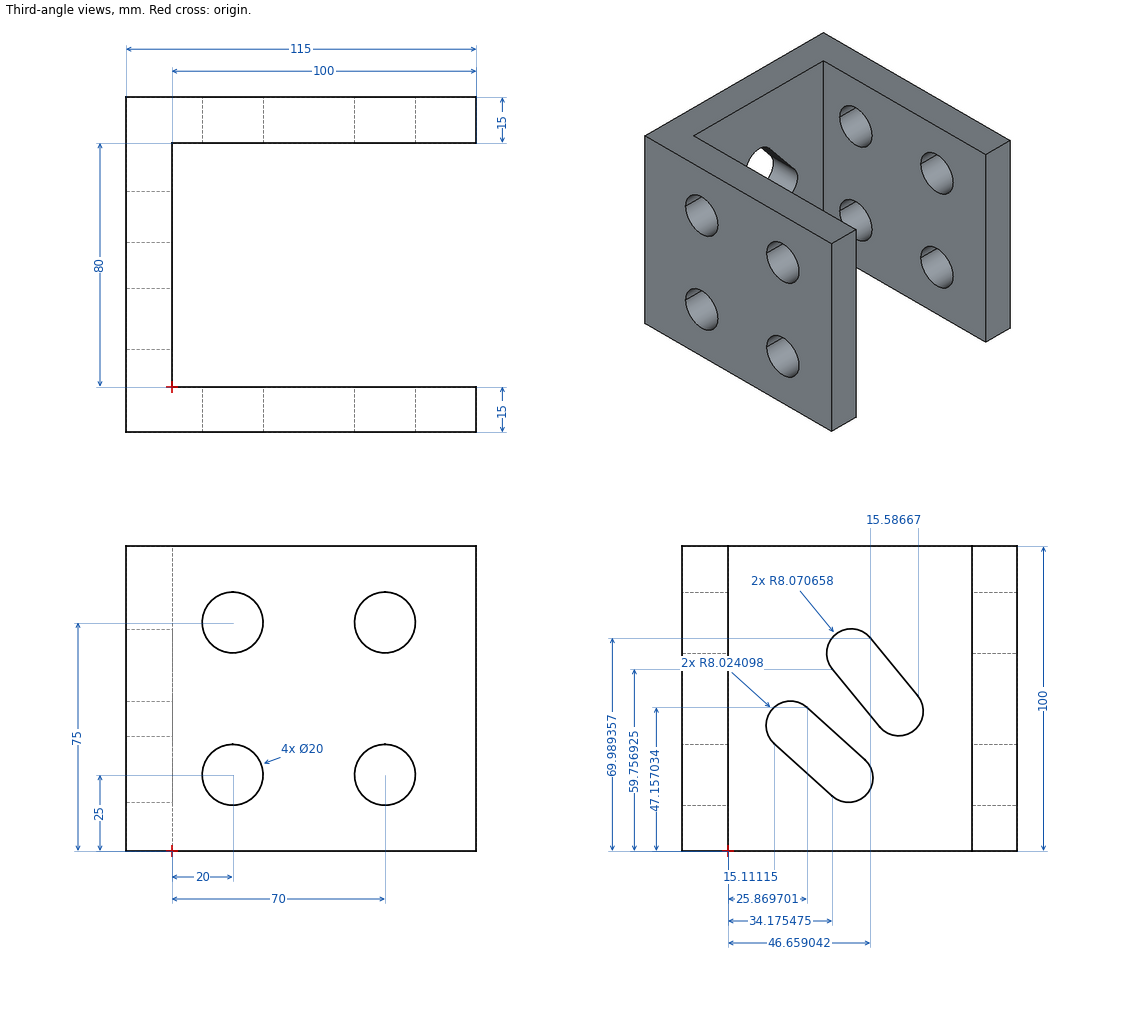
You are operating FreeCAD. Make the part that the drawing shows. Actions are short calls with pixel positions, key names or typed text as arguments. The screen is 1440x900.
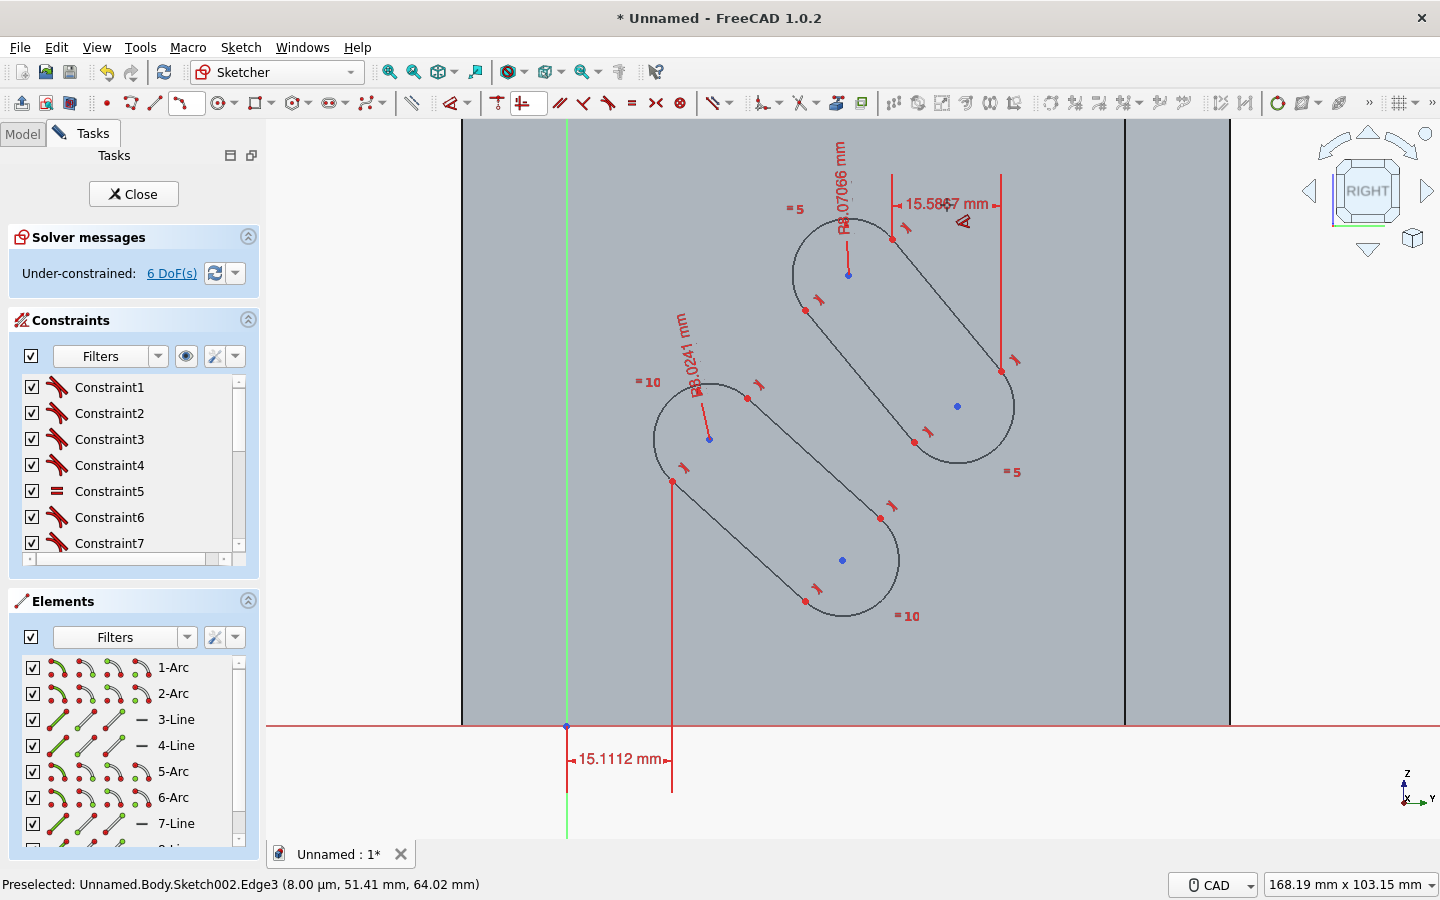
click(892, 239)
click(730, 760)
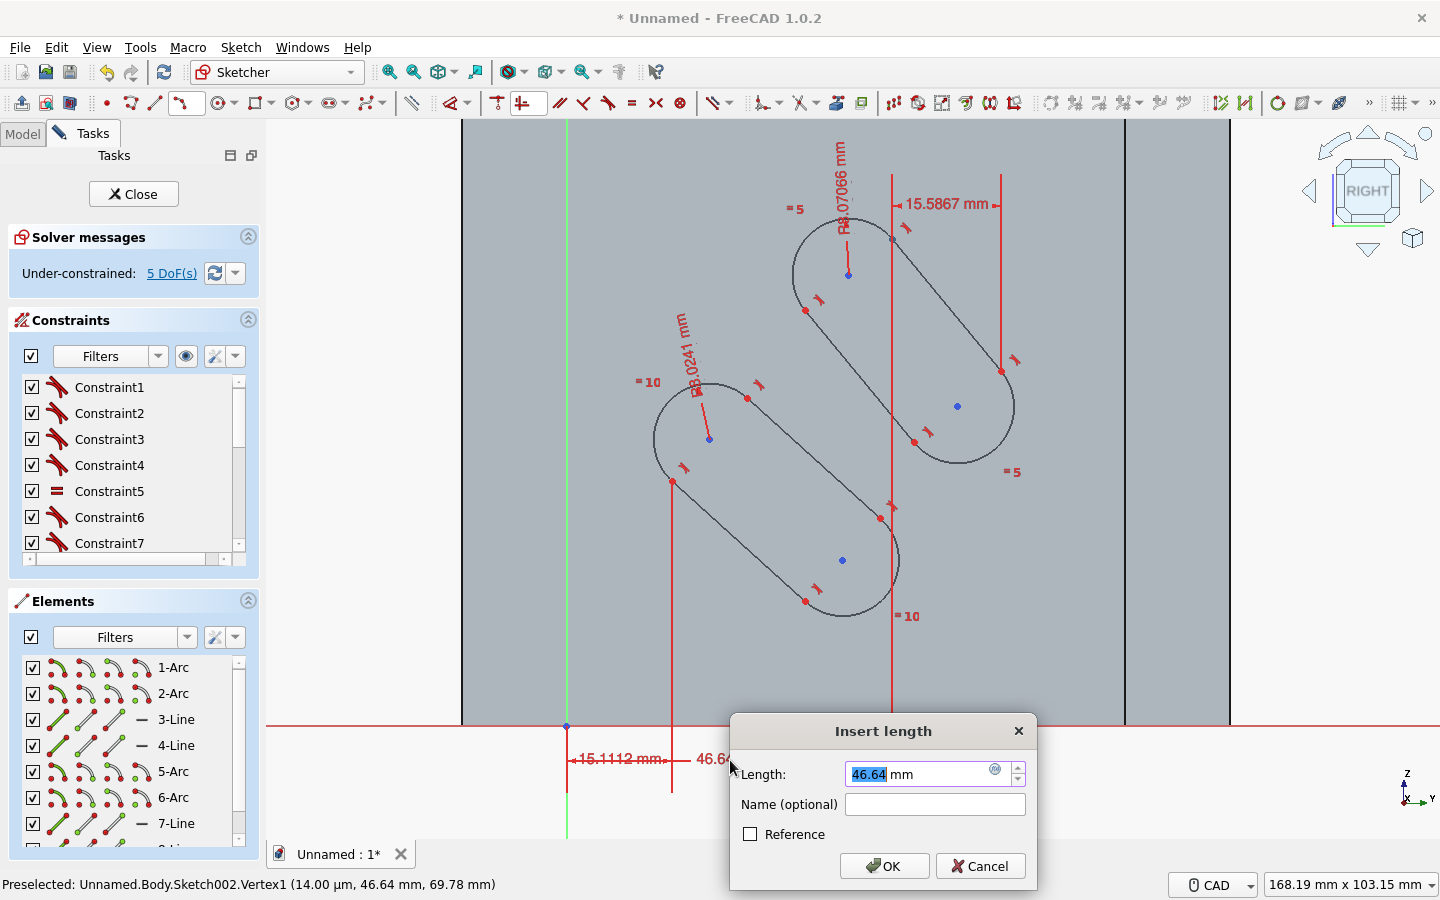
text(46.659042)
key(Return)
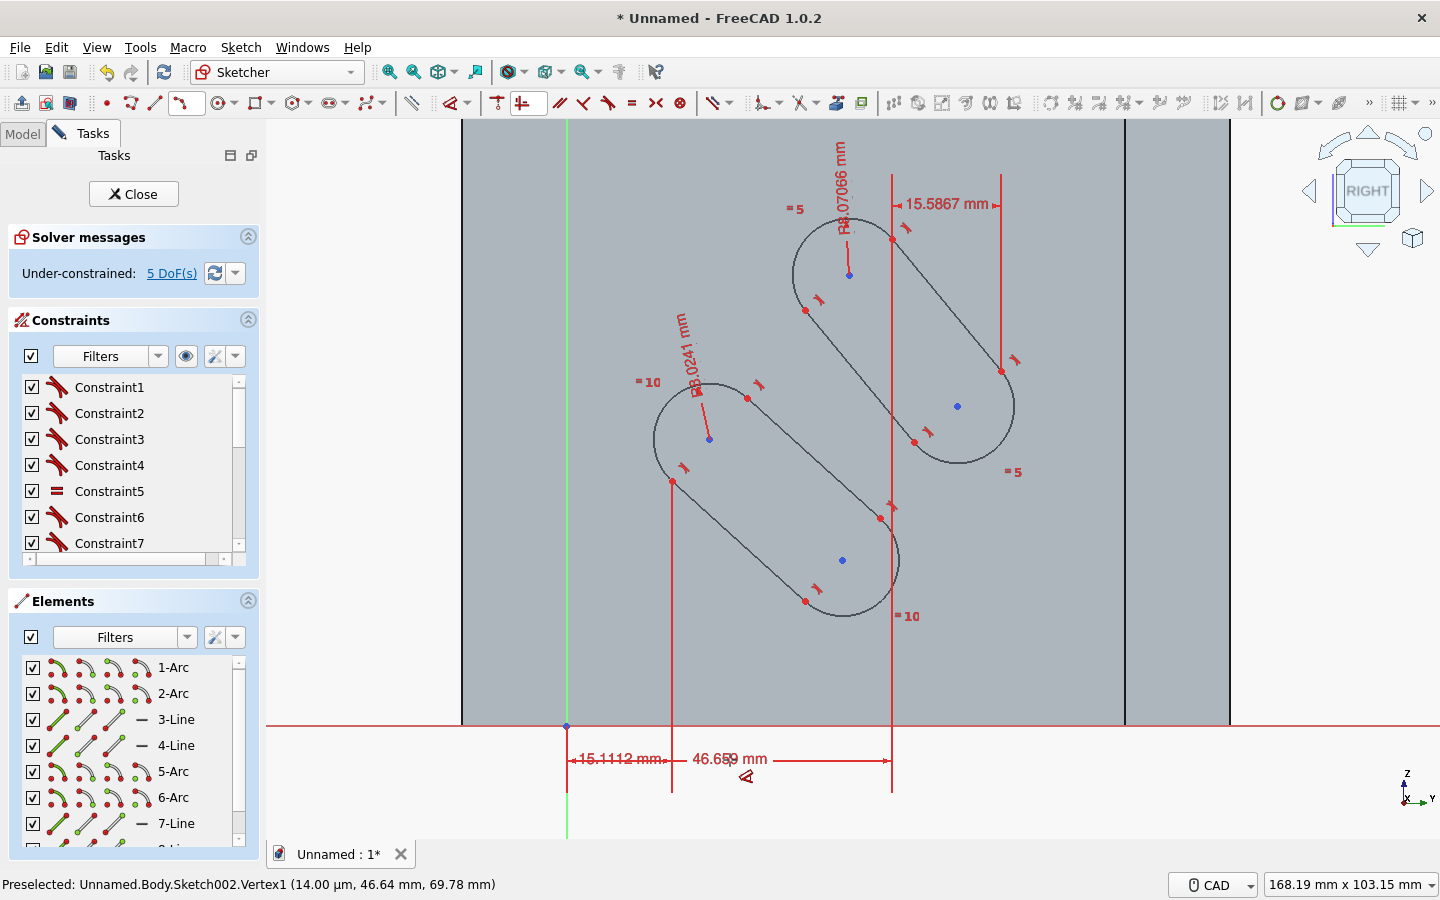
click(892, 239)
click(533, 483)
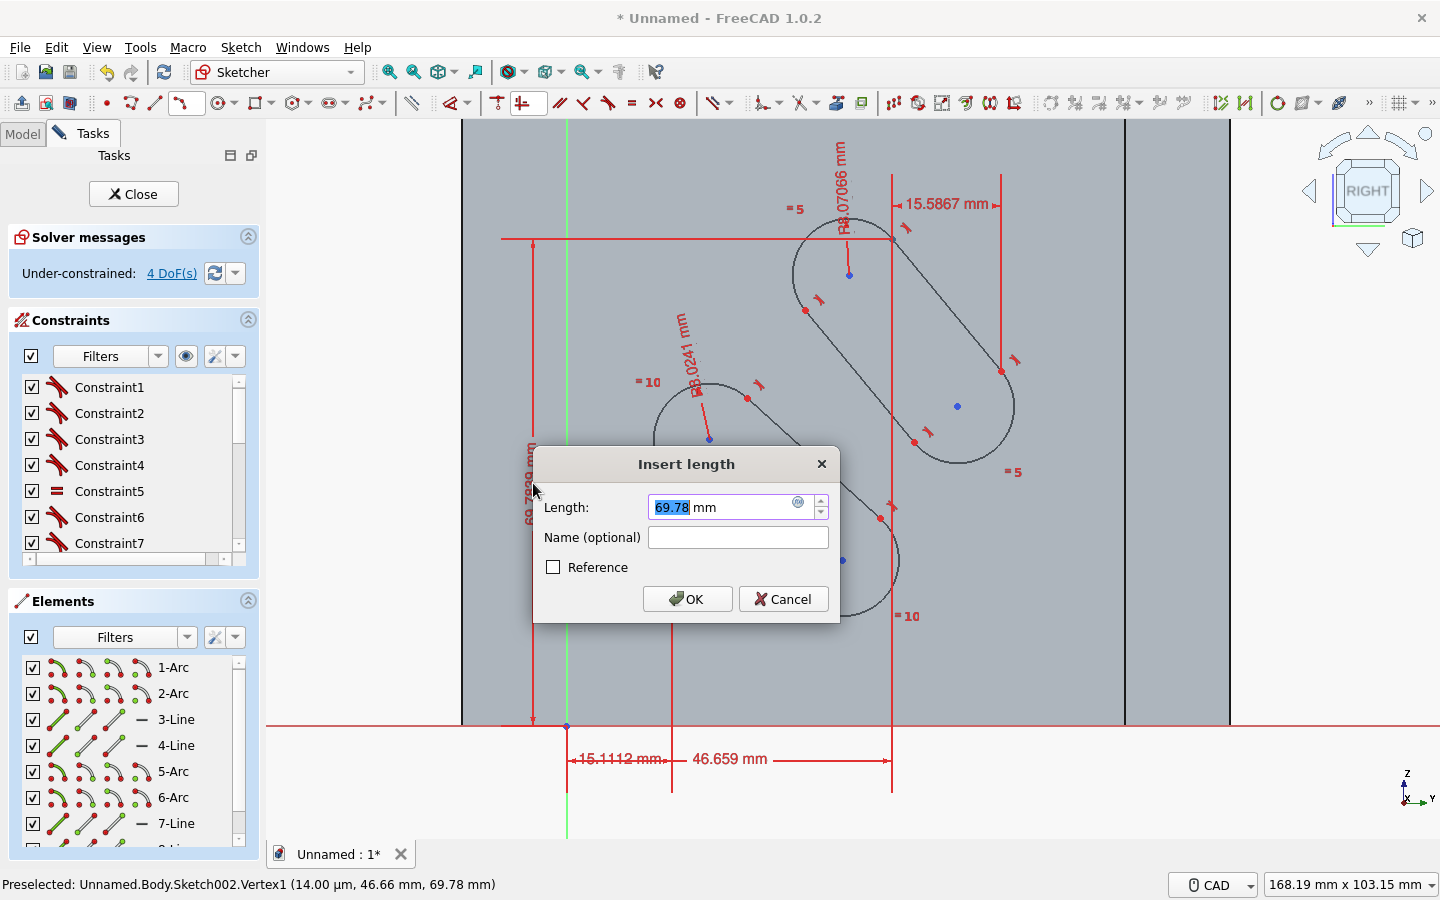
text(69.989357)
key(Return)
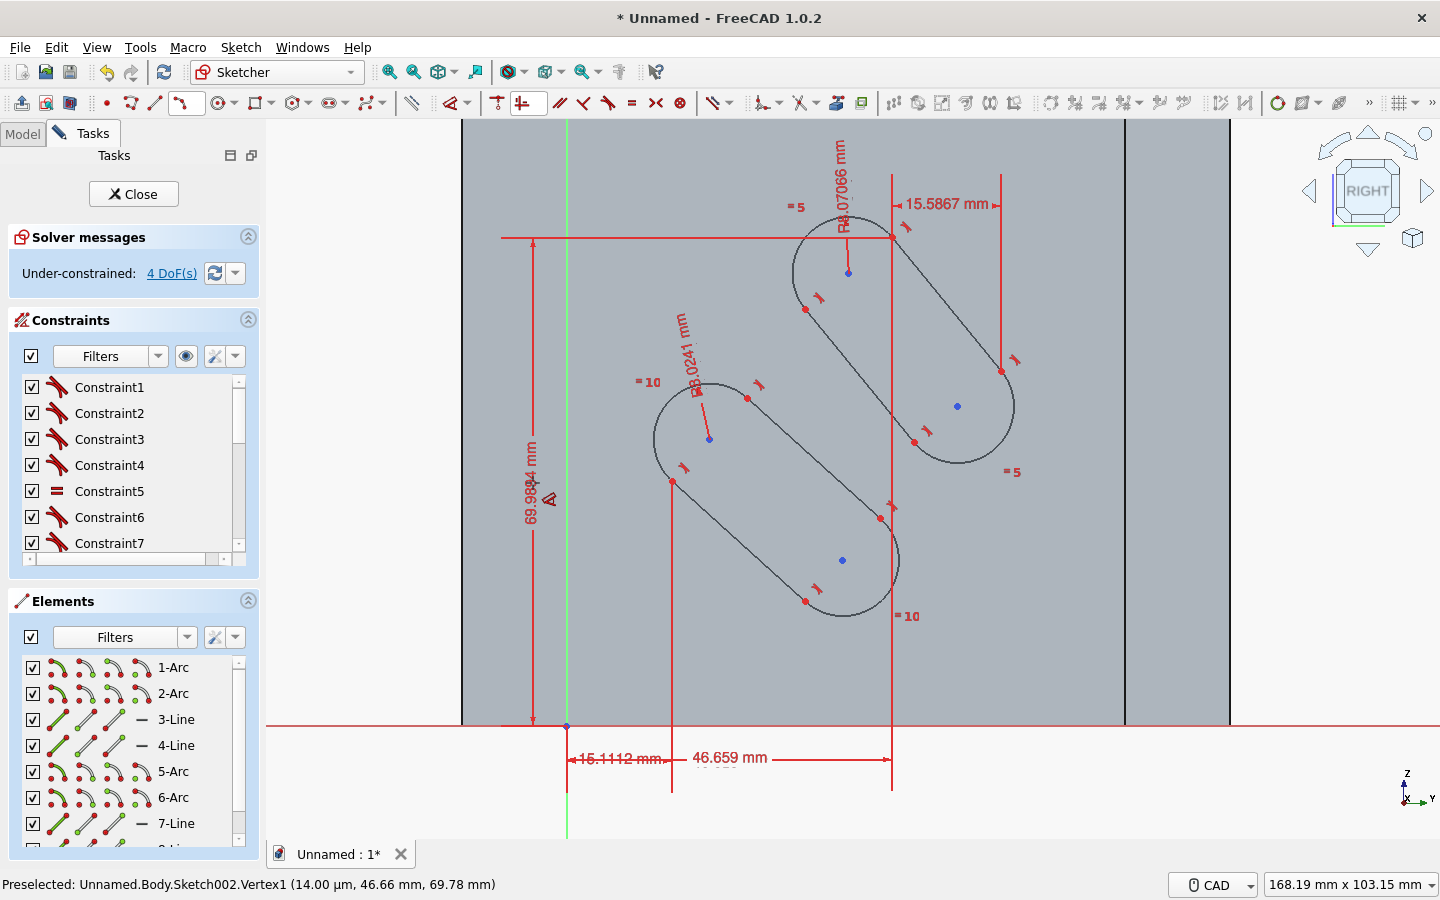
click(805, 309)
click(533, 518)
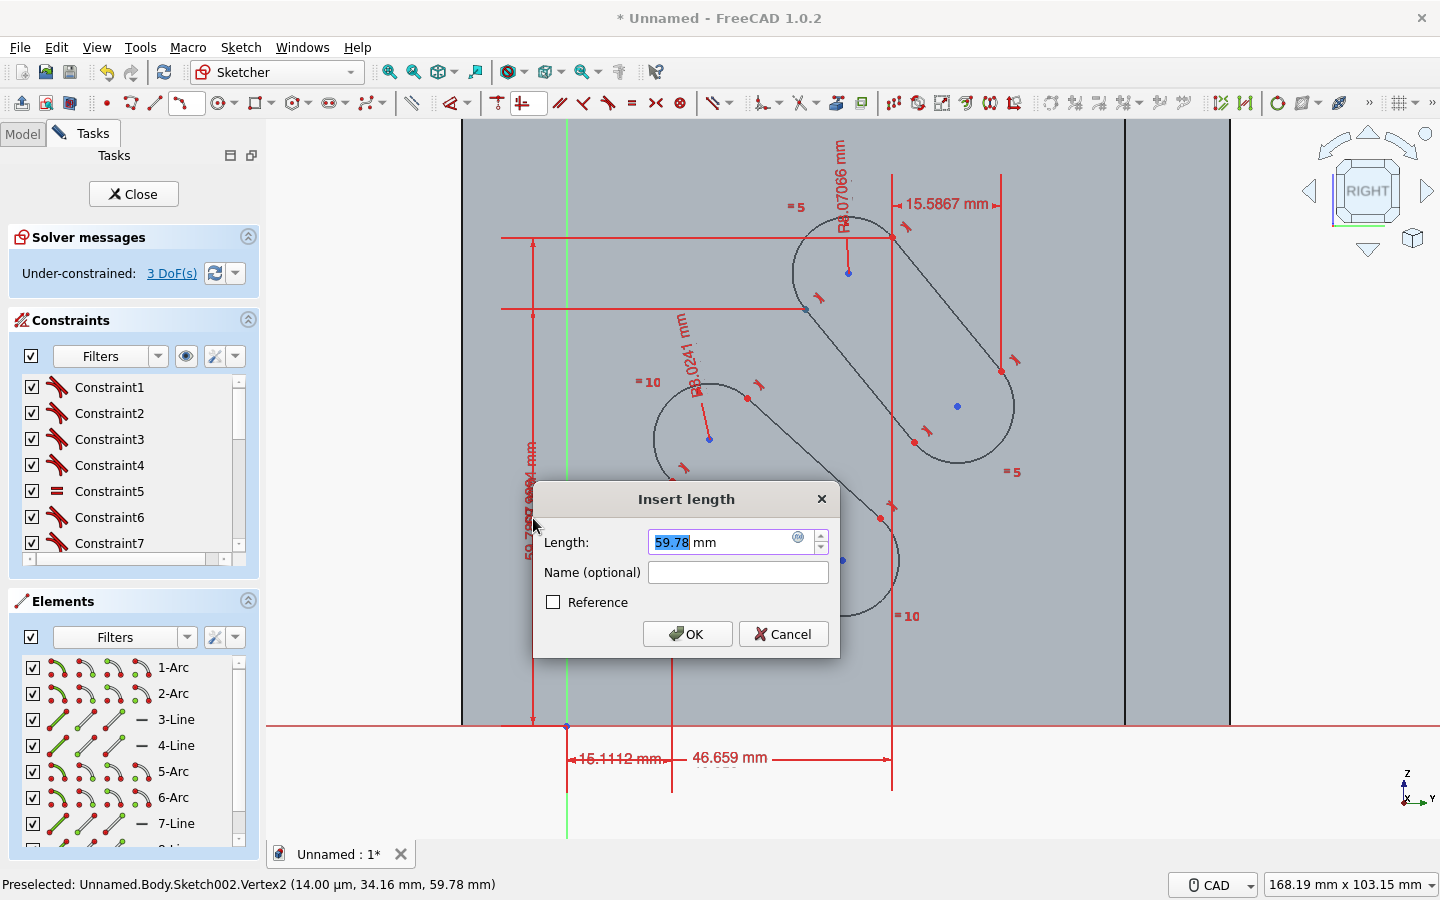
text(59.756925)
key(Return)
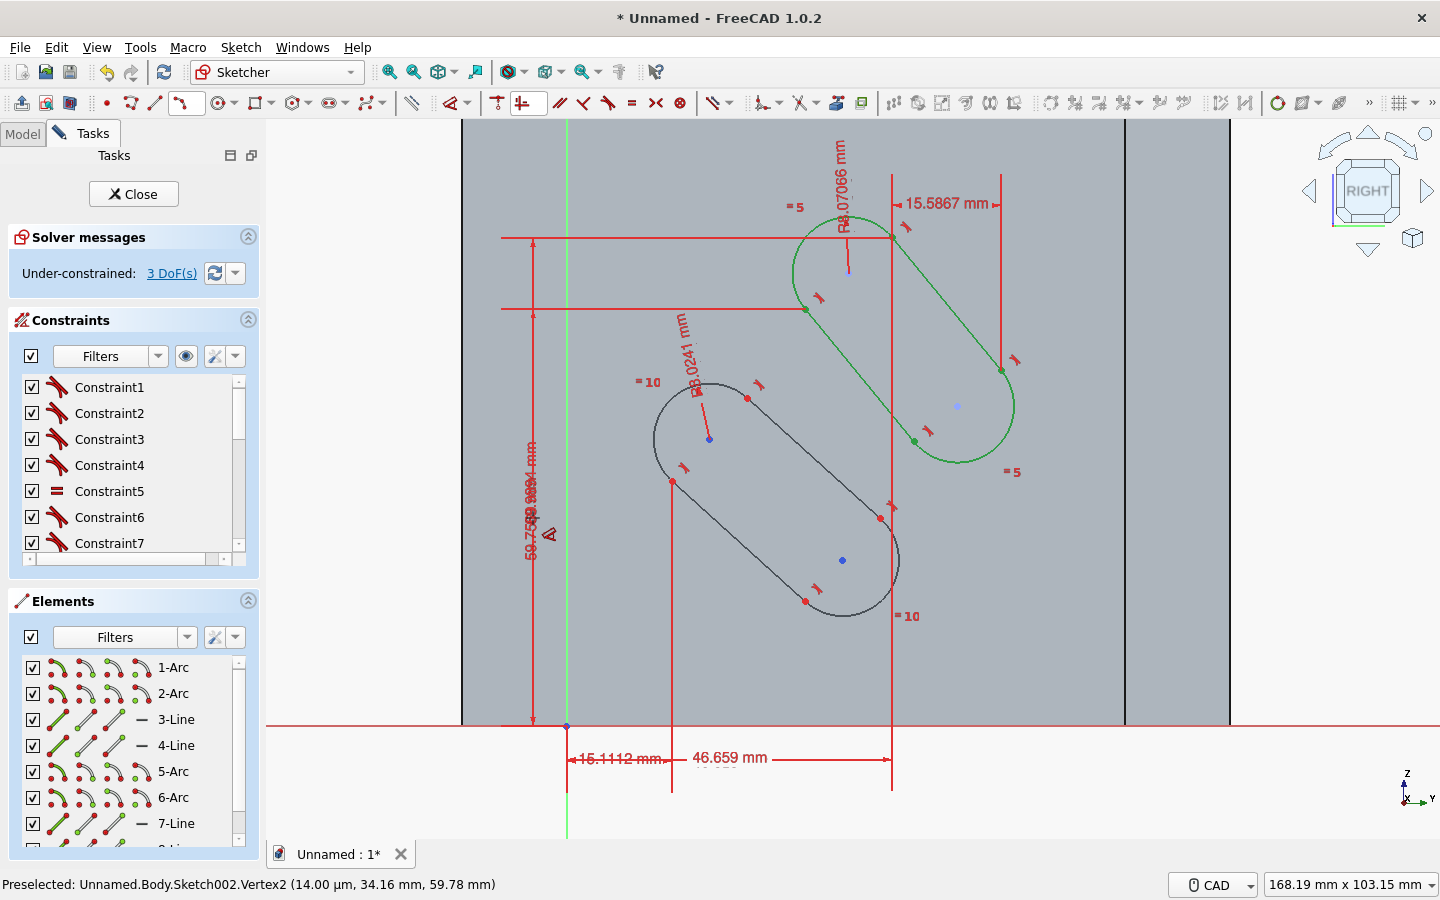
click(747, 398)
click(616, 364)